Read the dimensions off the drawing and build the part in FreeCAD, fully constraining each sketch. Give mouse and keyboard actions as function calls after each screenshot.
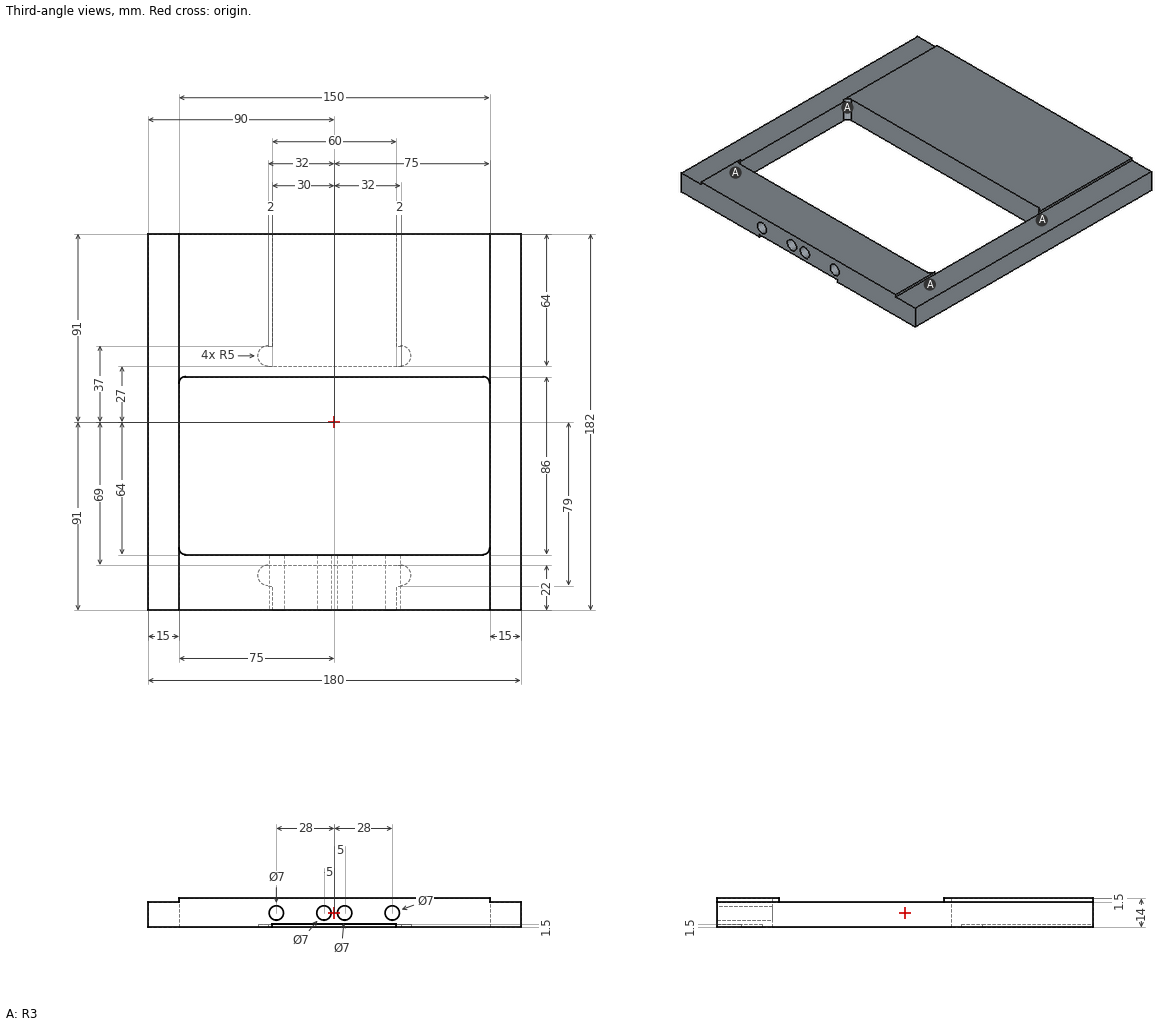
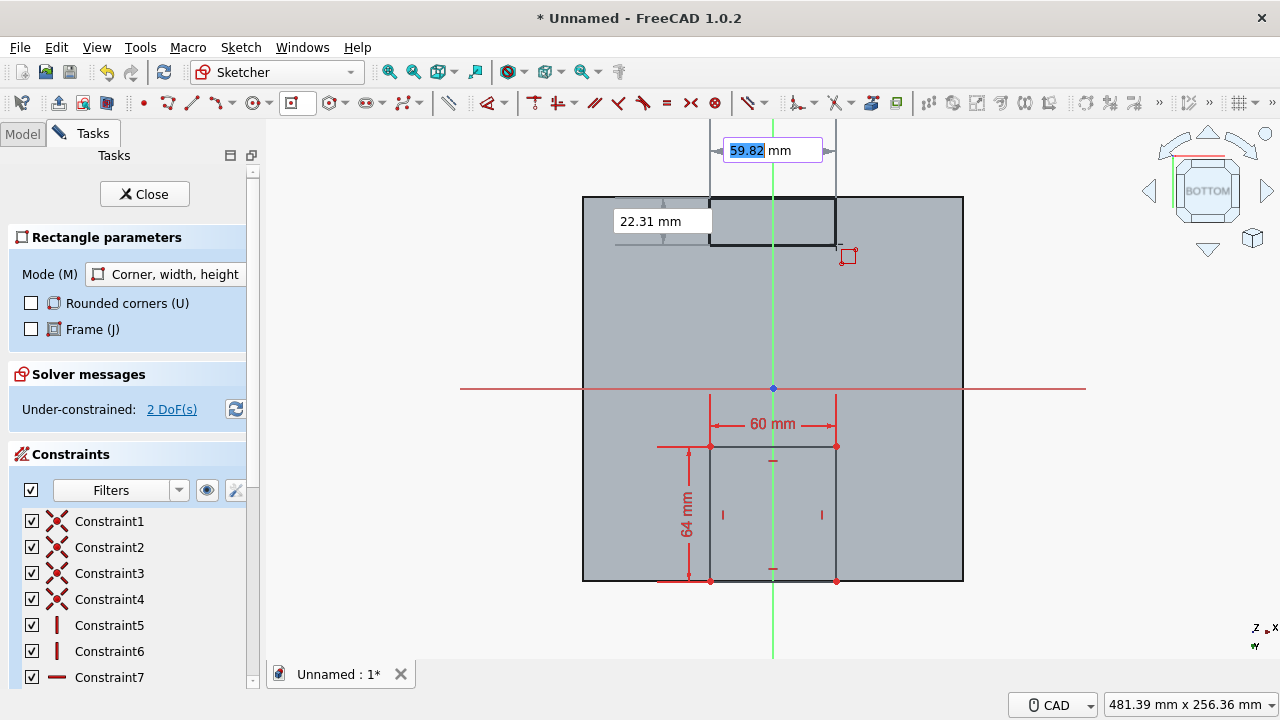
text(60)
key(Tab)
text(22)
key(Return)
key(Escape)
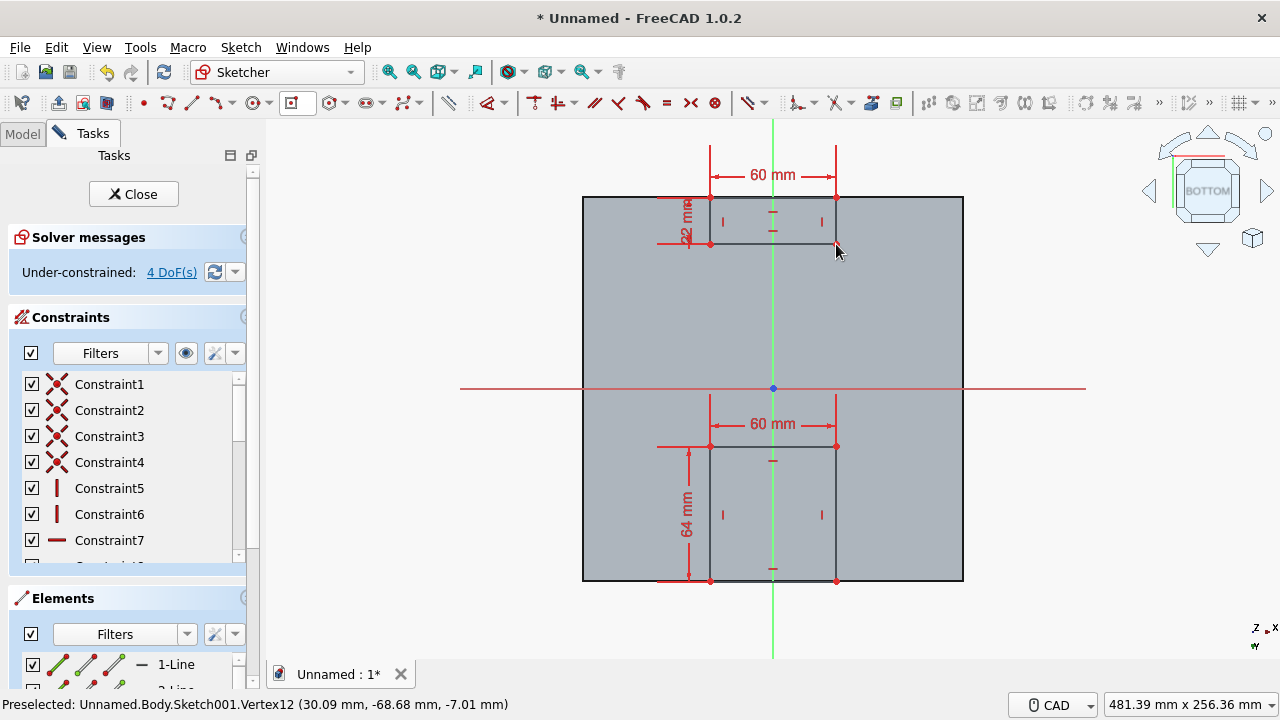
click(710, 447)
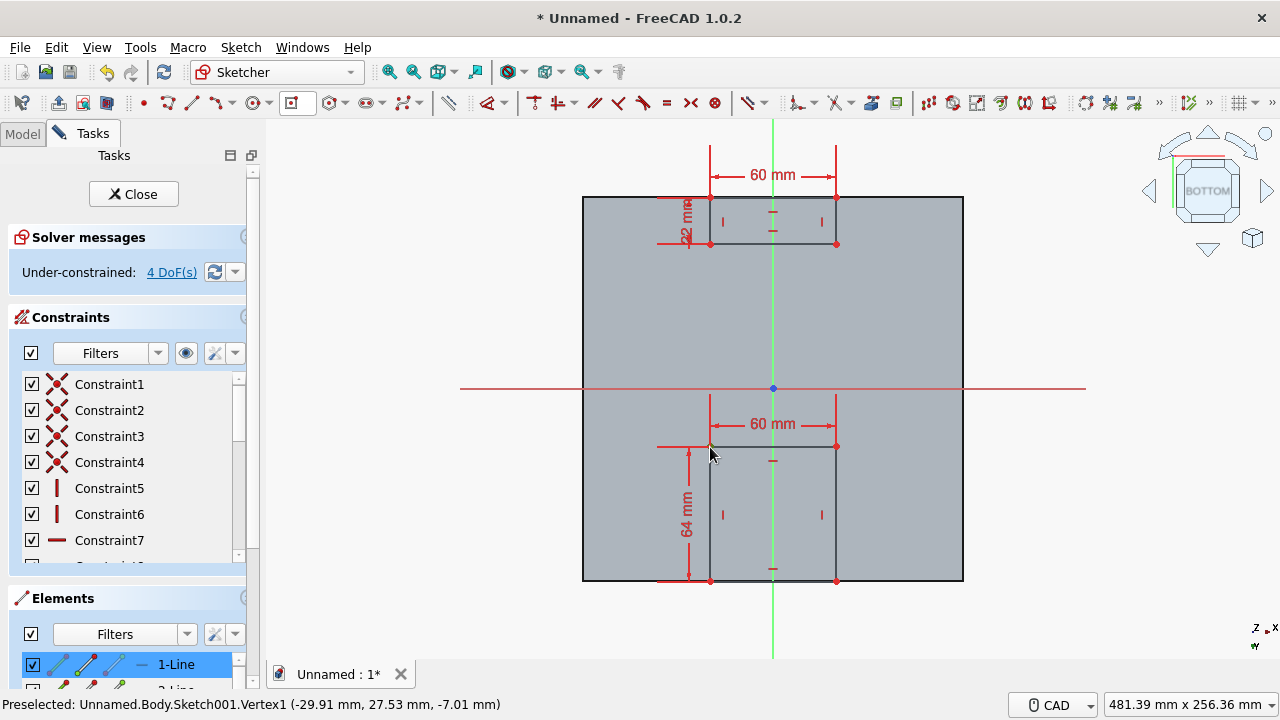
key(l)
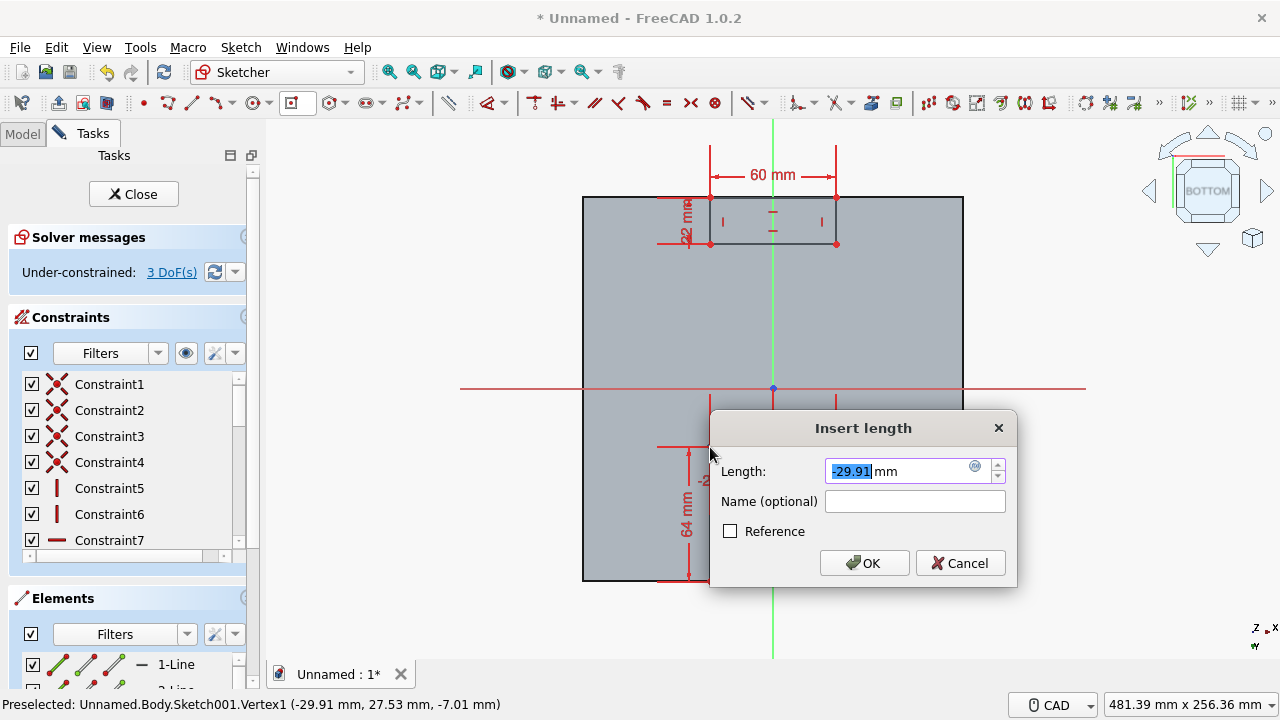
text(-30)
key(Return)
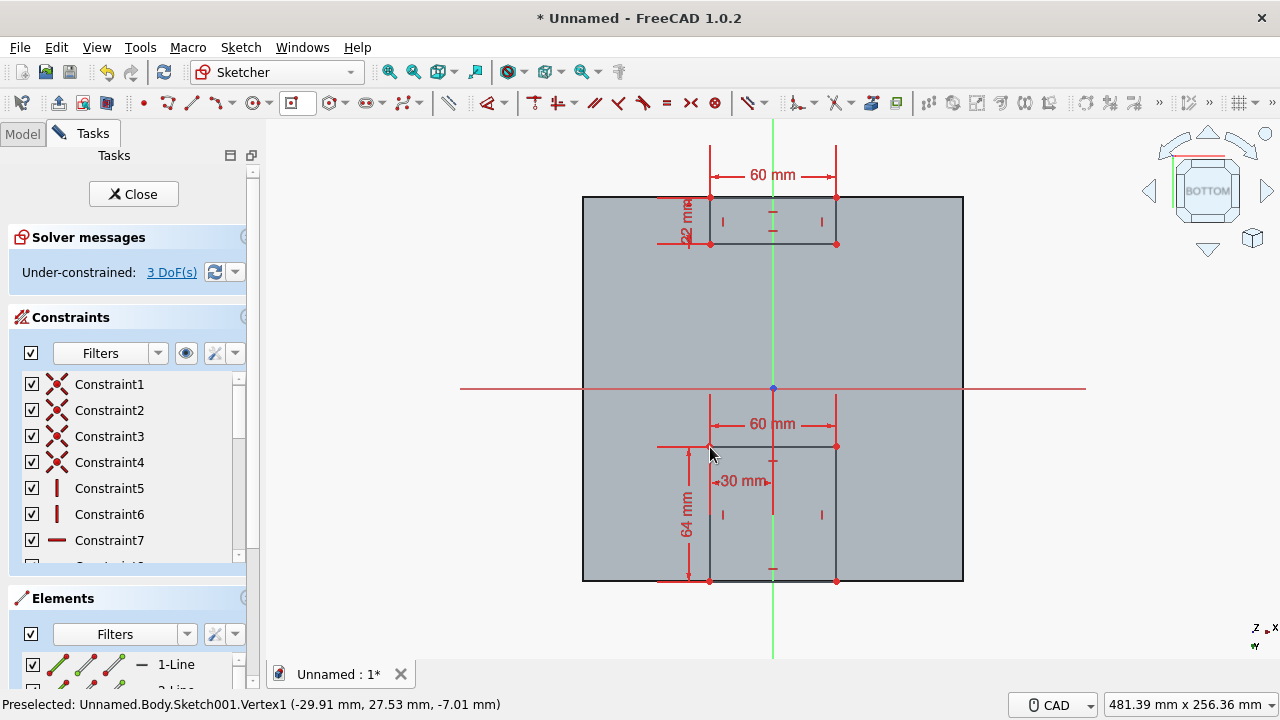
click(710, 447)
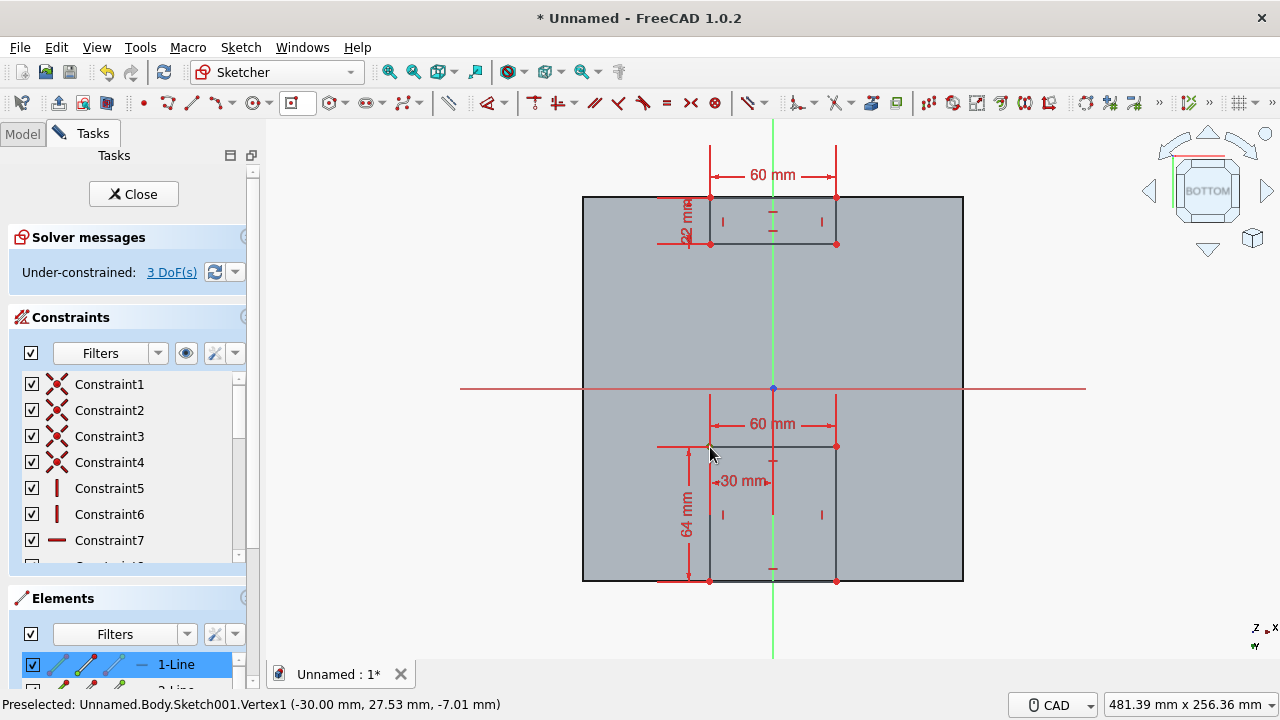
key(i)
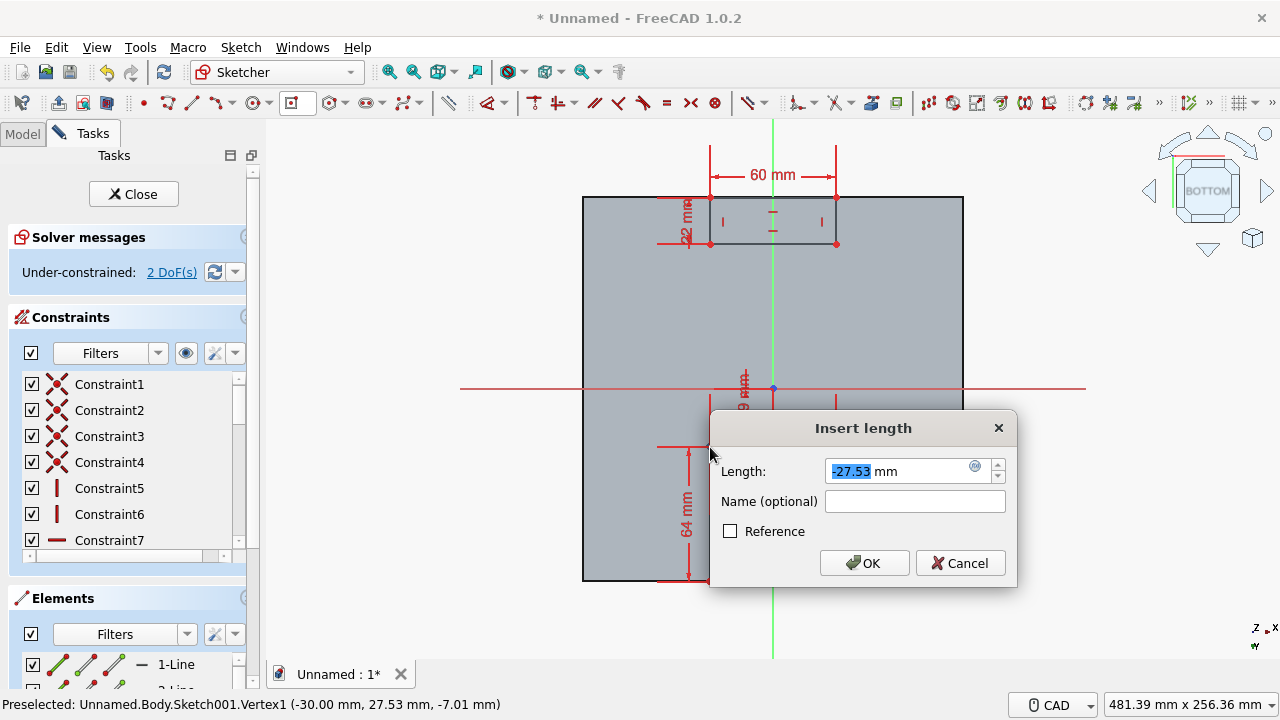
text(-27)
key(Return)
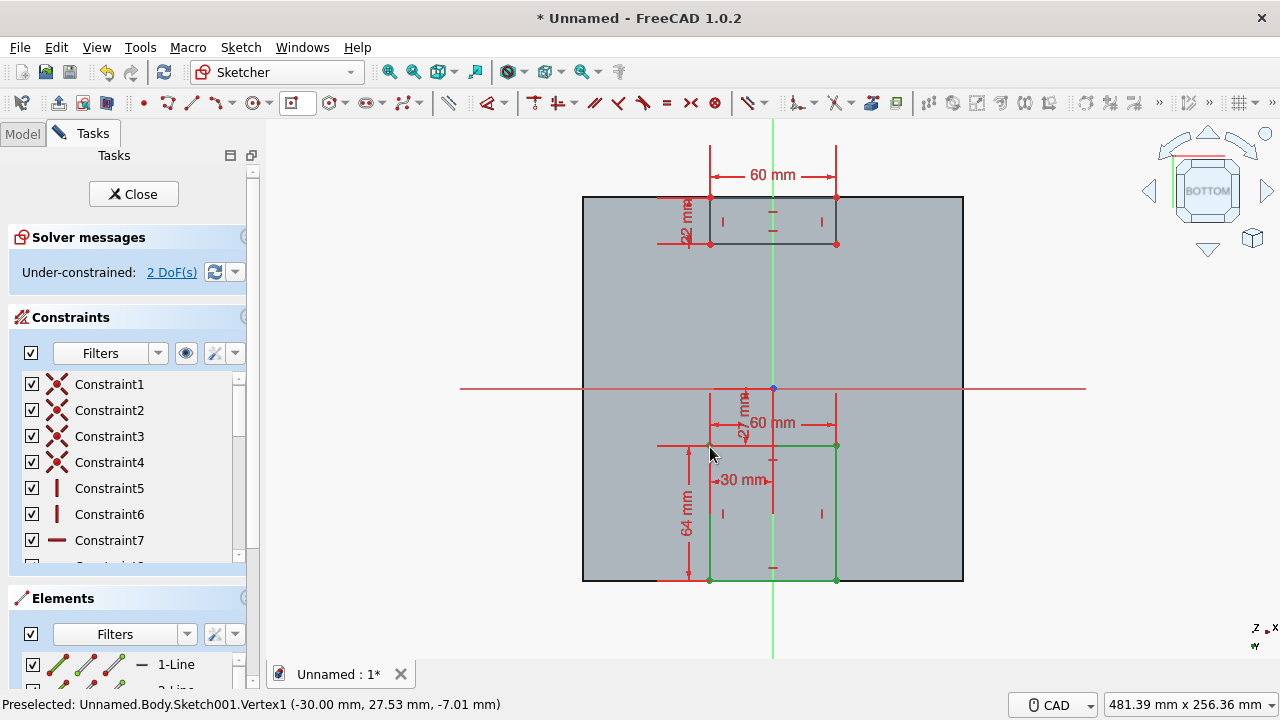
click(710, 198)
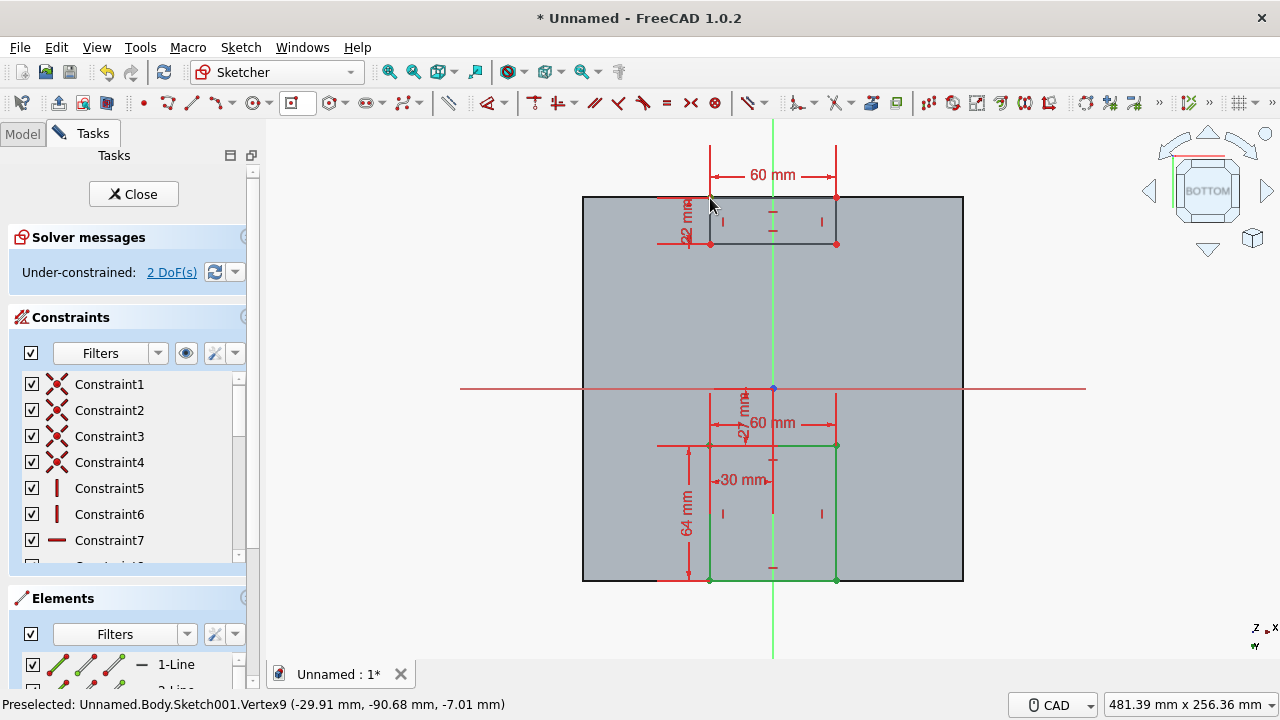
key(l)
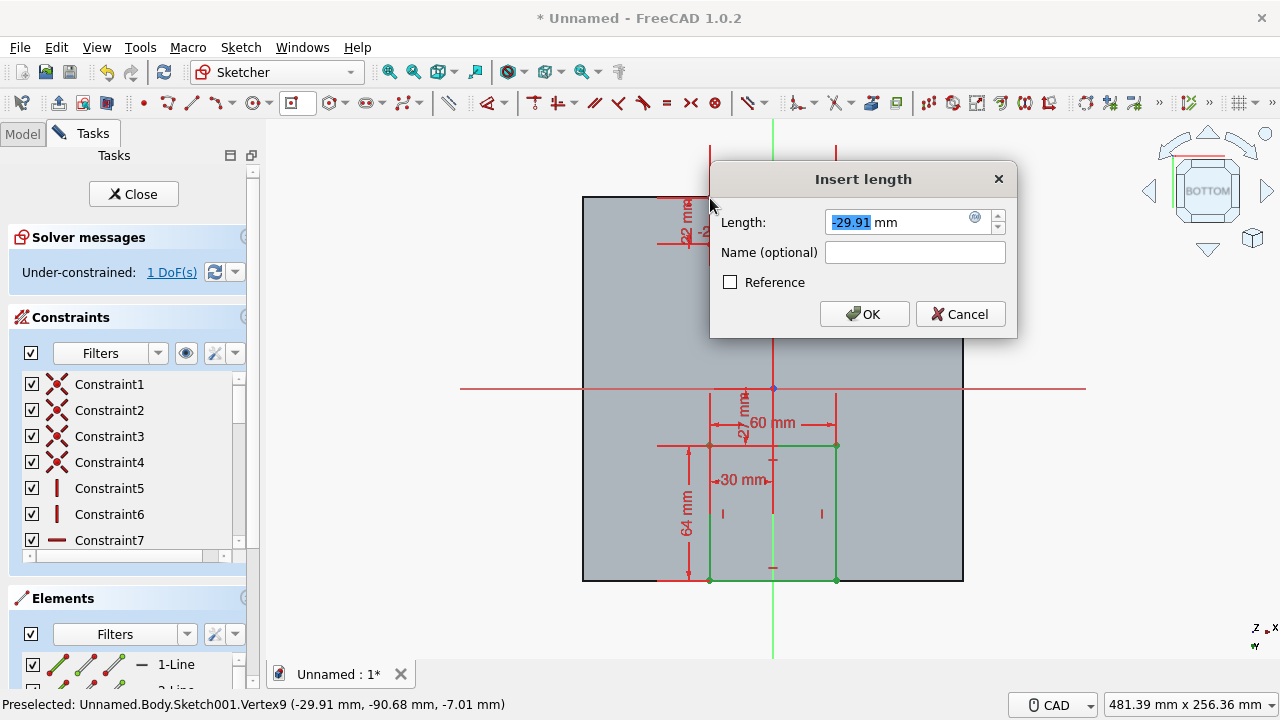
text(-30)
key(Return)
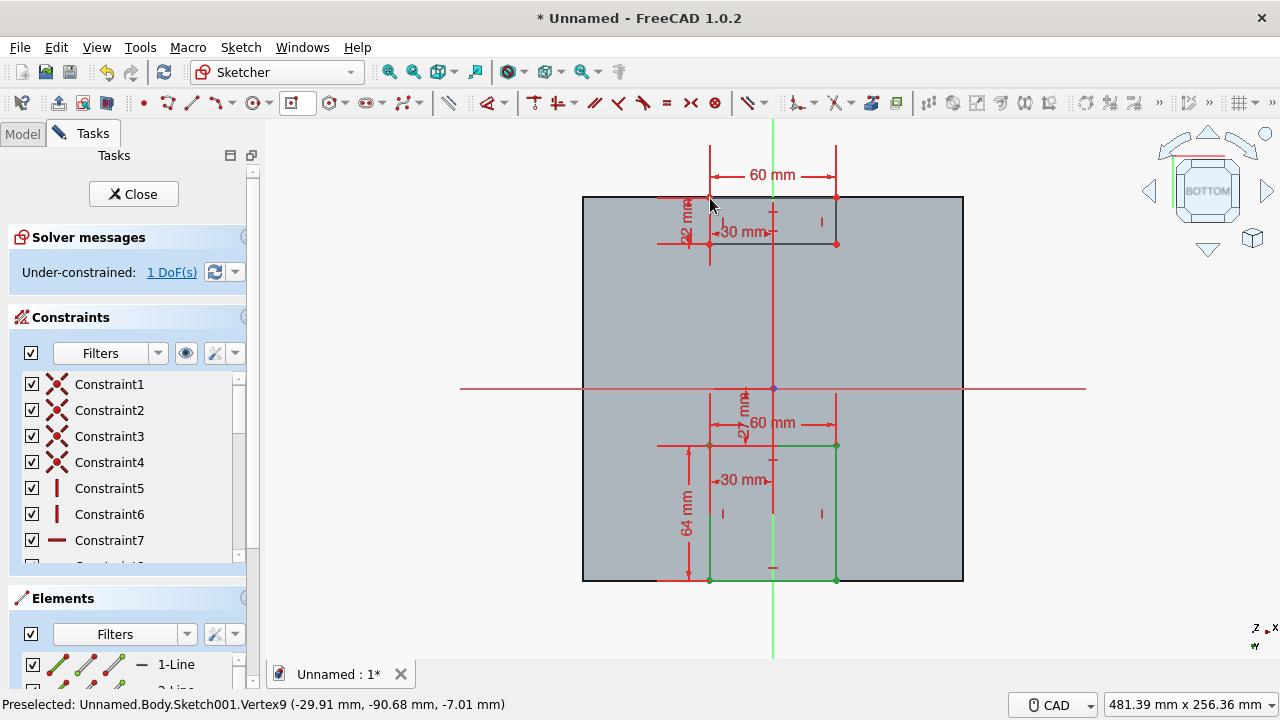
click(710, 198)